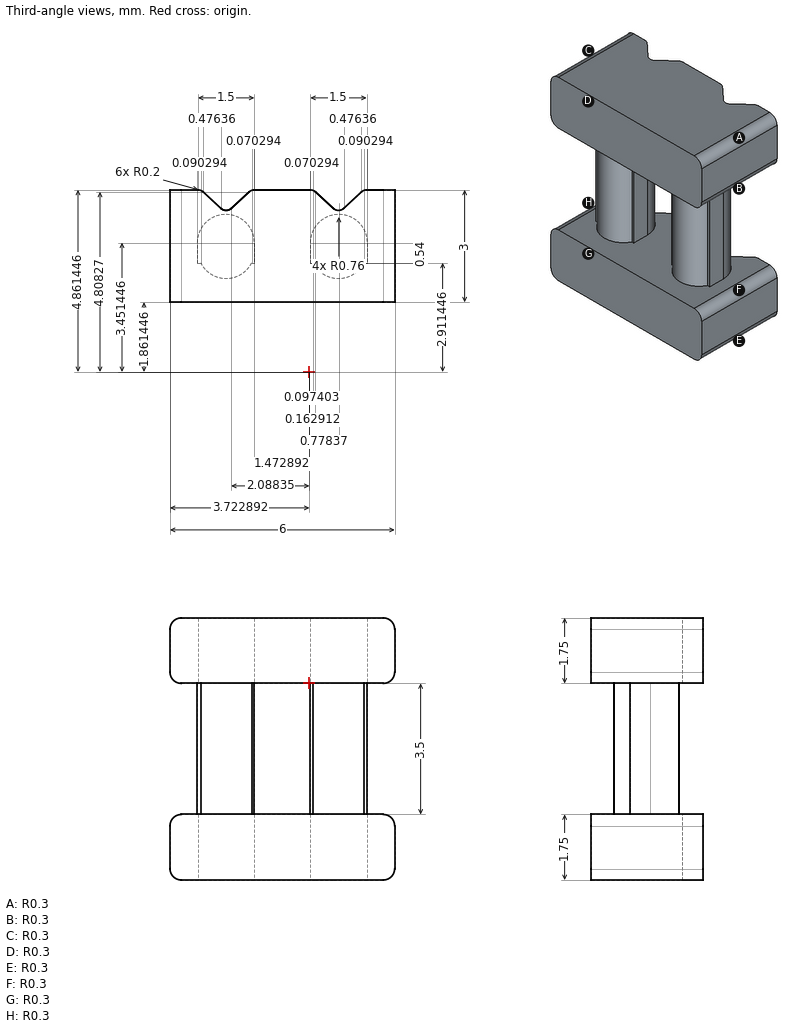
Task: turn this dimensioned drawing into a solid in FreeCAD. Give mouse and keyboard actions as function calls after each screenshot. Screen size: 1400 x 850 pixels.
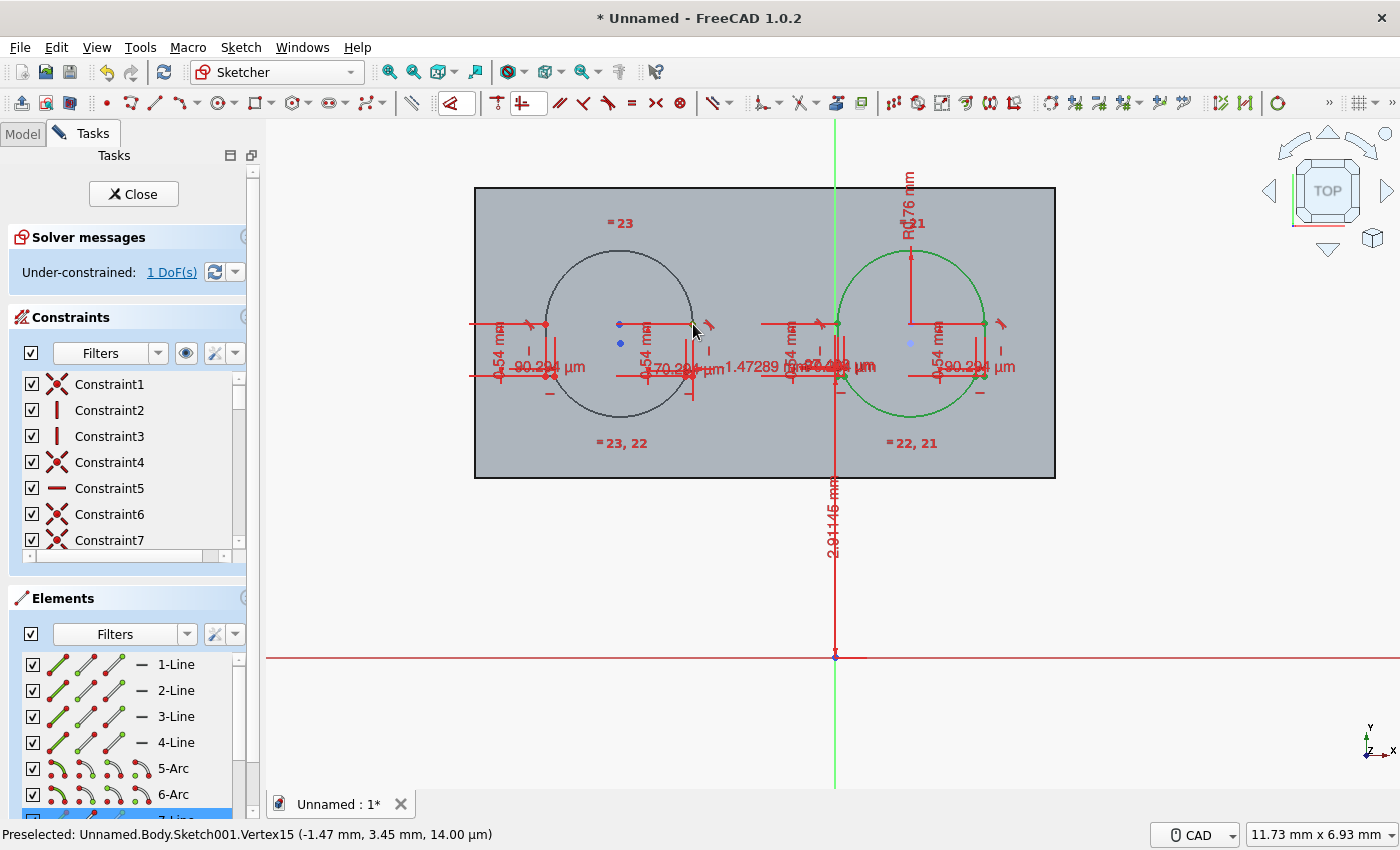
key(i)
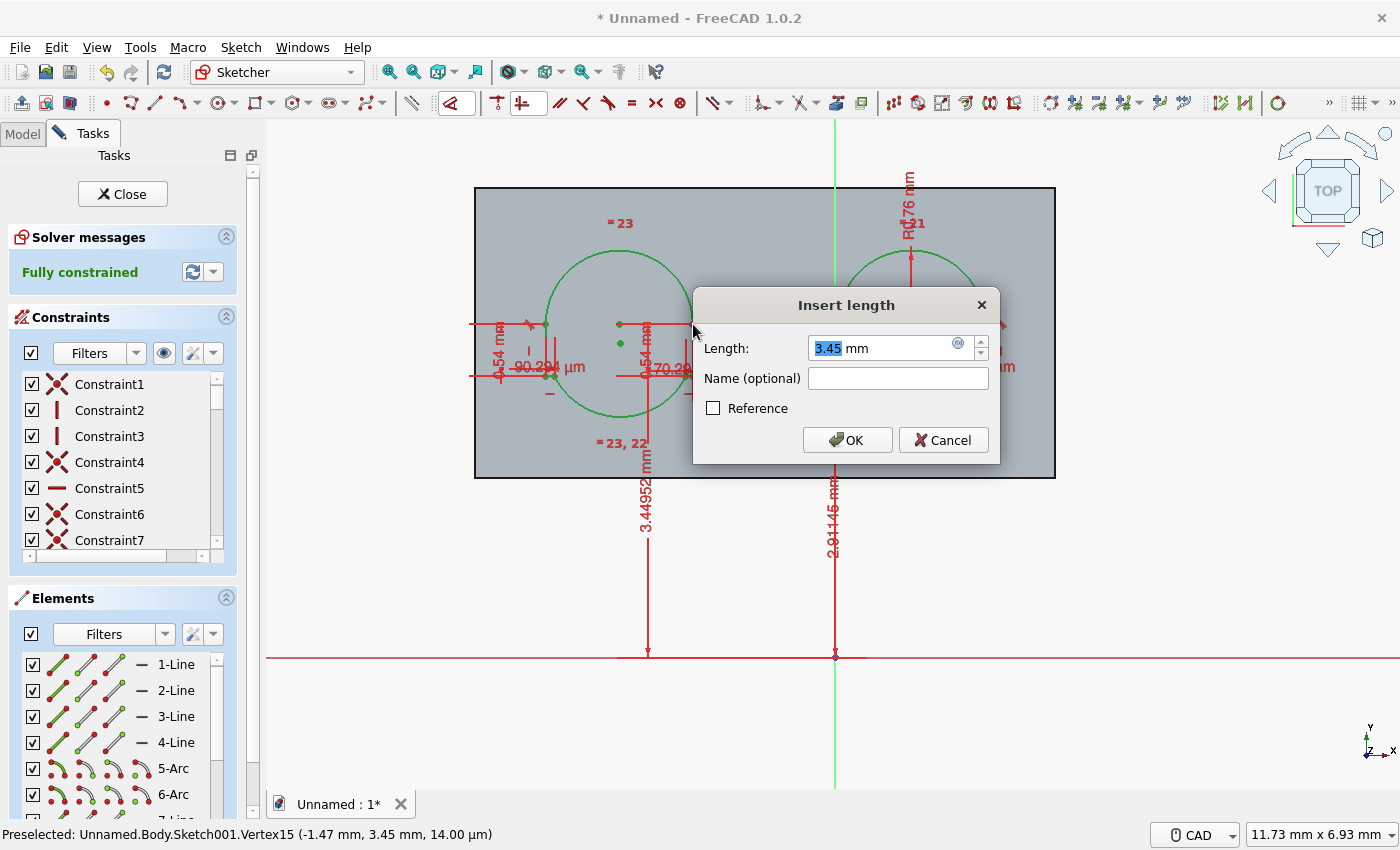
text(3.451446)
key(Return)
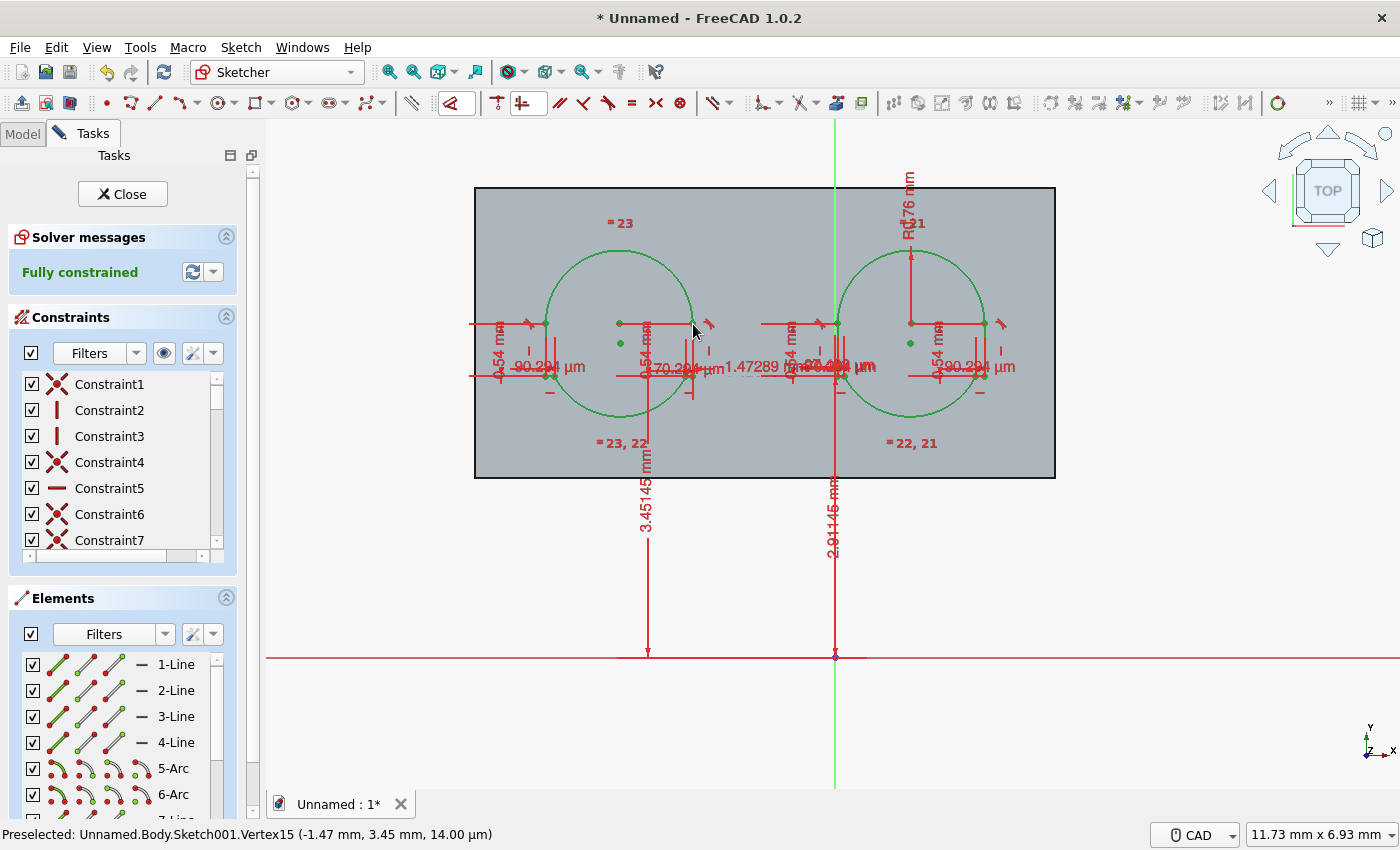
click(123, 194)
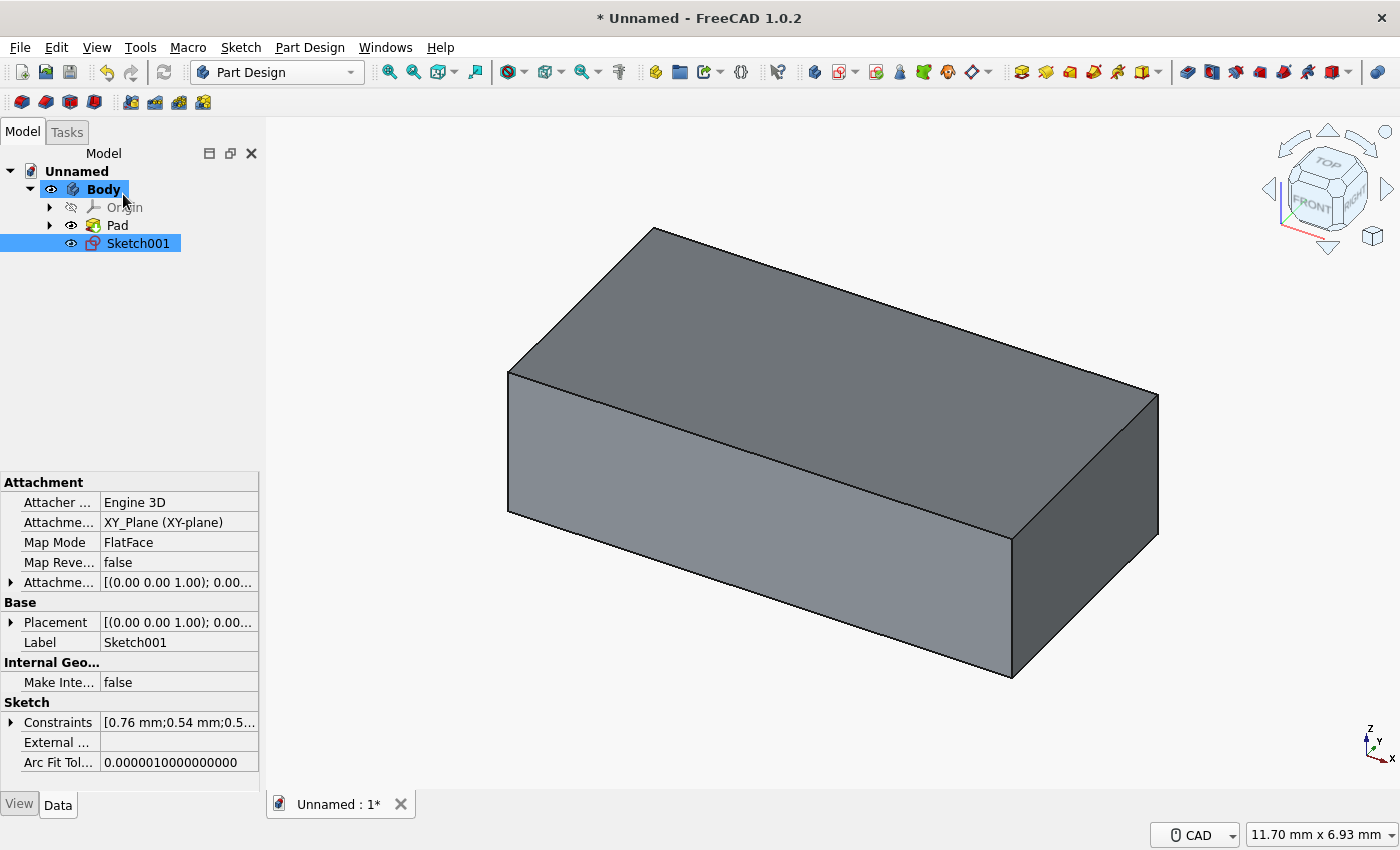
click(1022, 72)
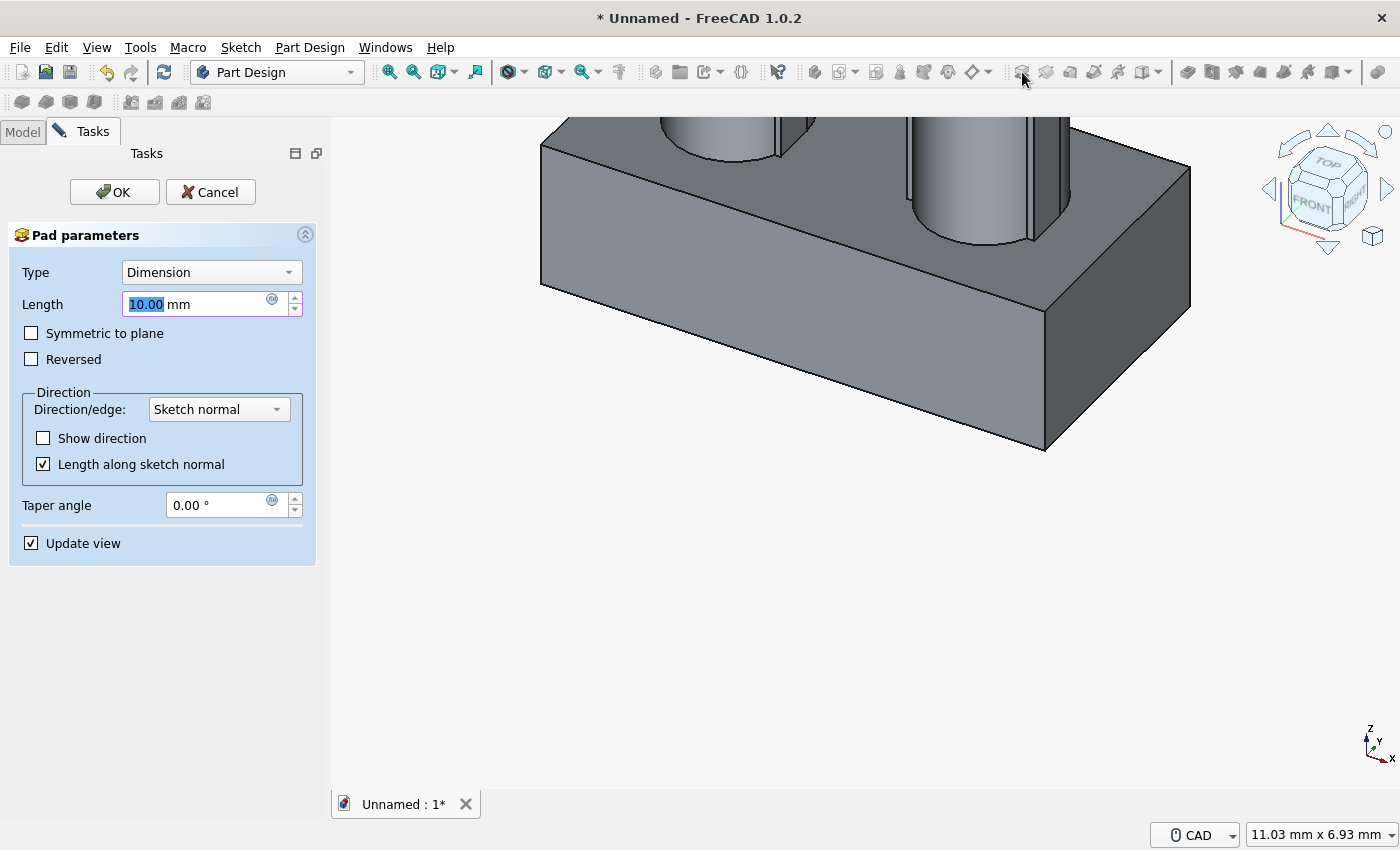
text(3.5)
key(Tab)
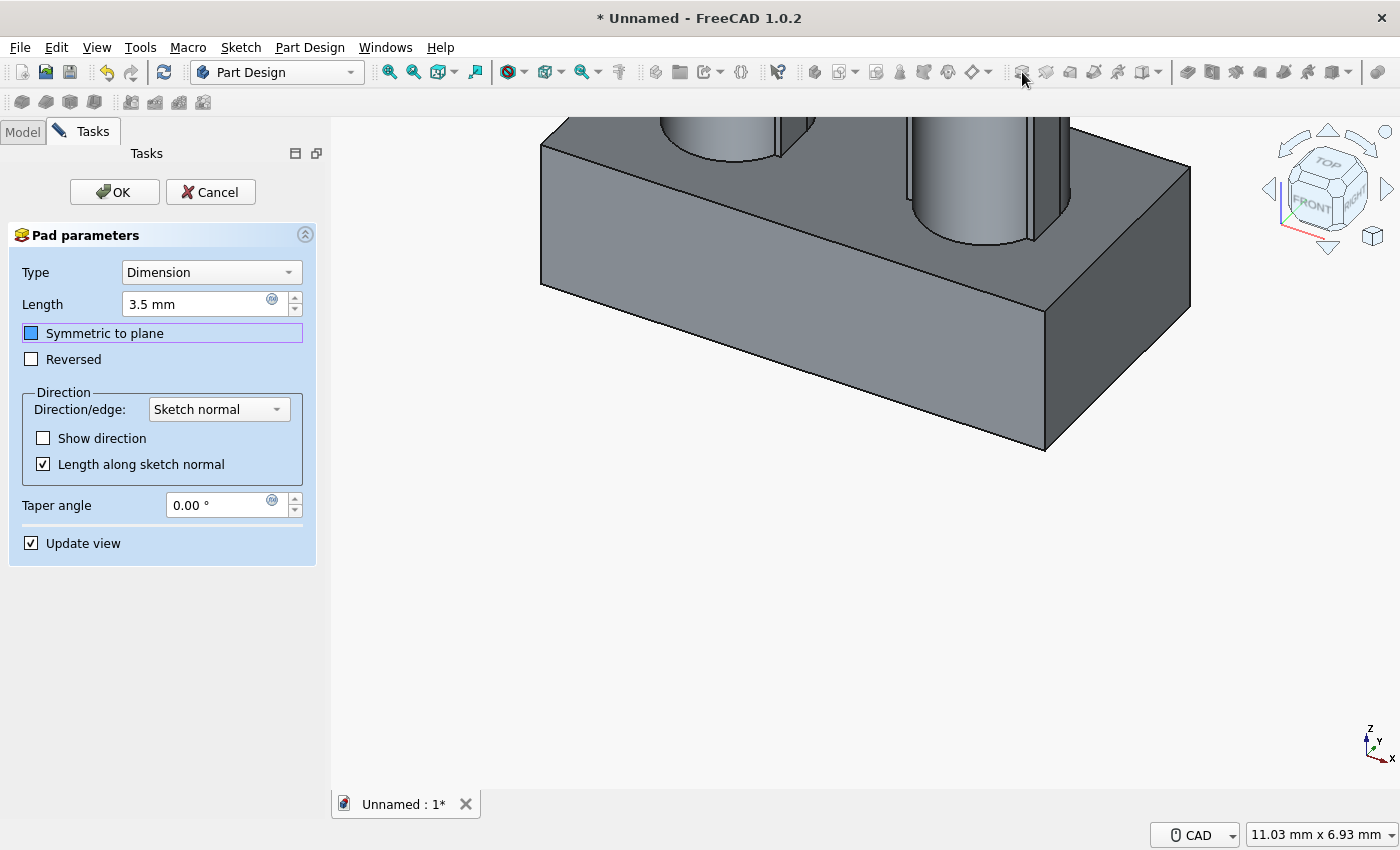
click(30, 359)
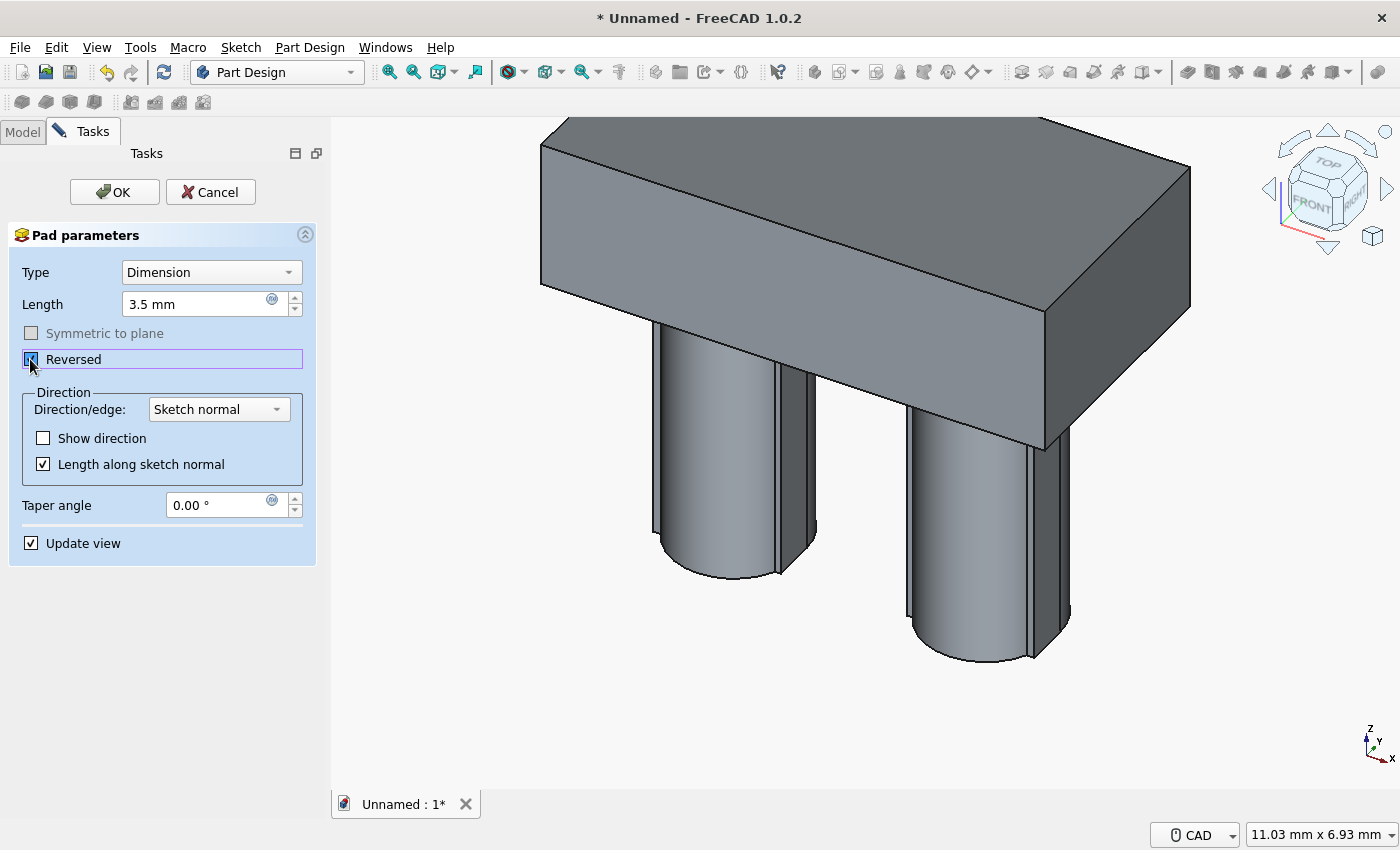
click(115, 192)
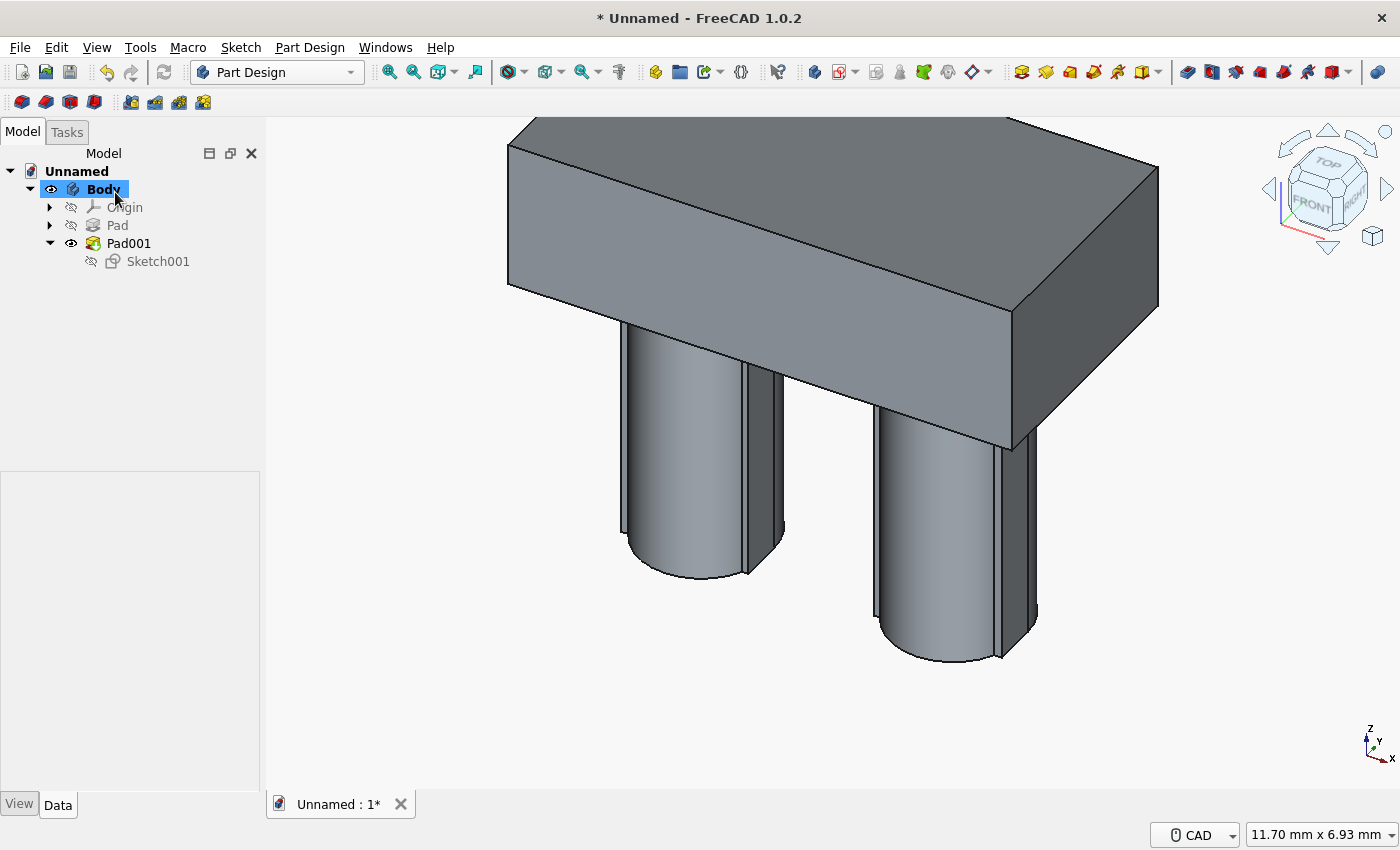
click(390, 72)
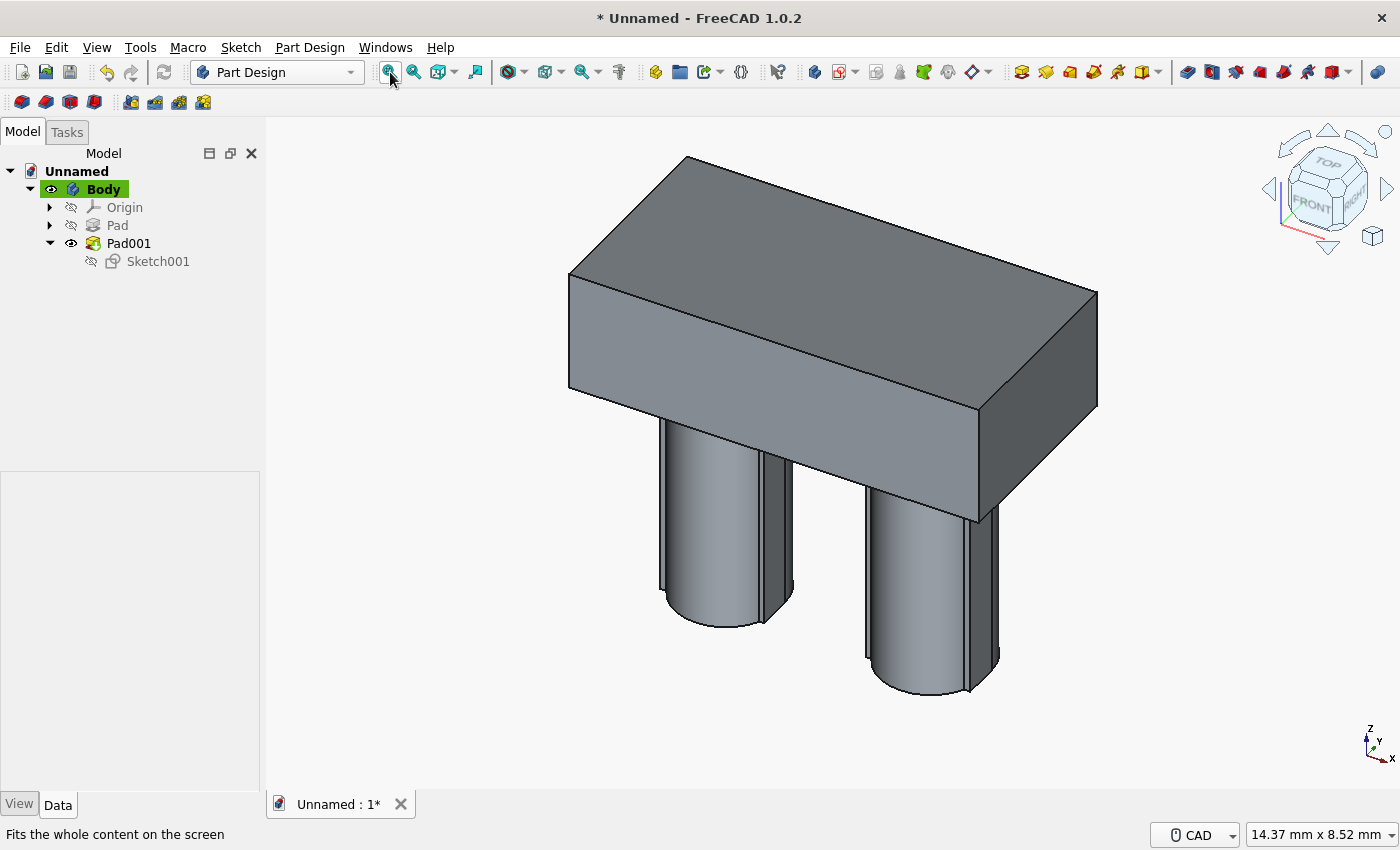
click(1038, 350)